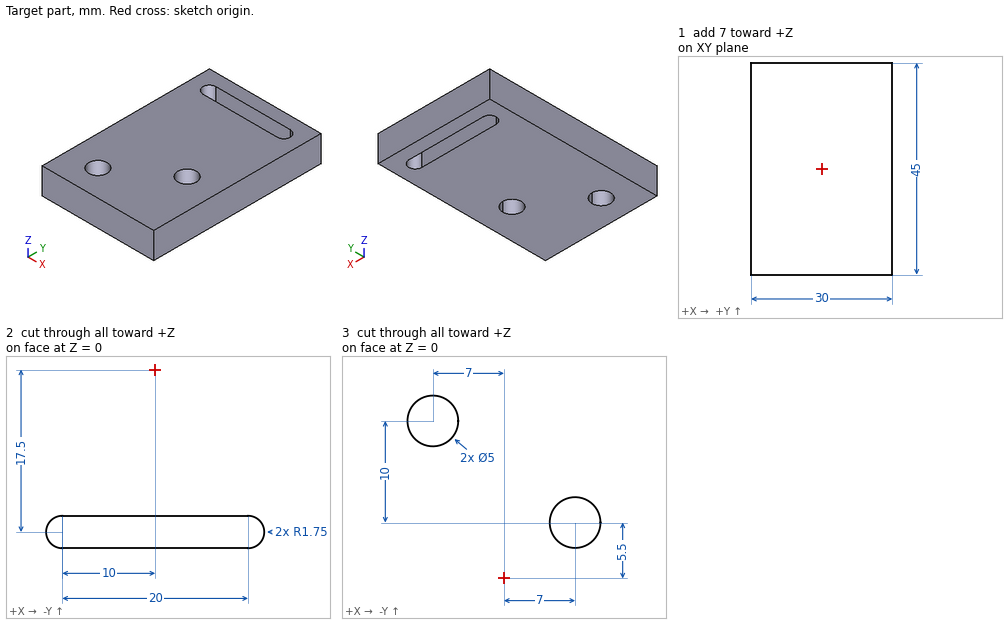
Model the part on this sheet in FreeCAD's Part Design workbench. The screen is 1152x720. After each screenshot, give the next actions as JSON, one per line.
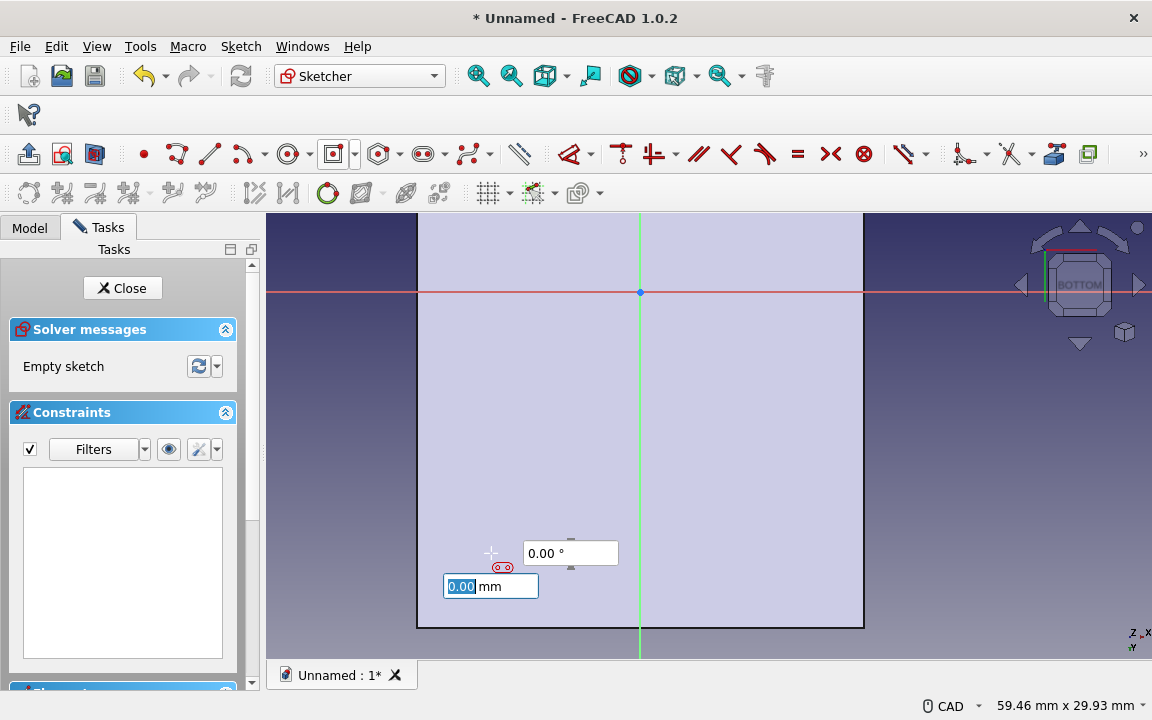
{"action": "left_click", "coordinate": [789, 553]}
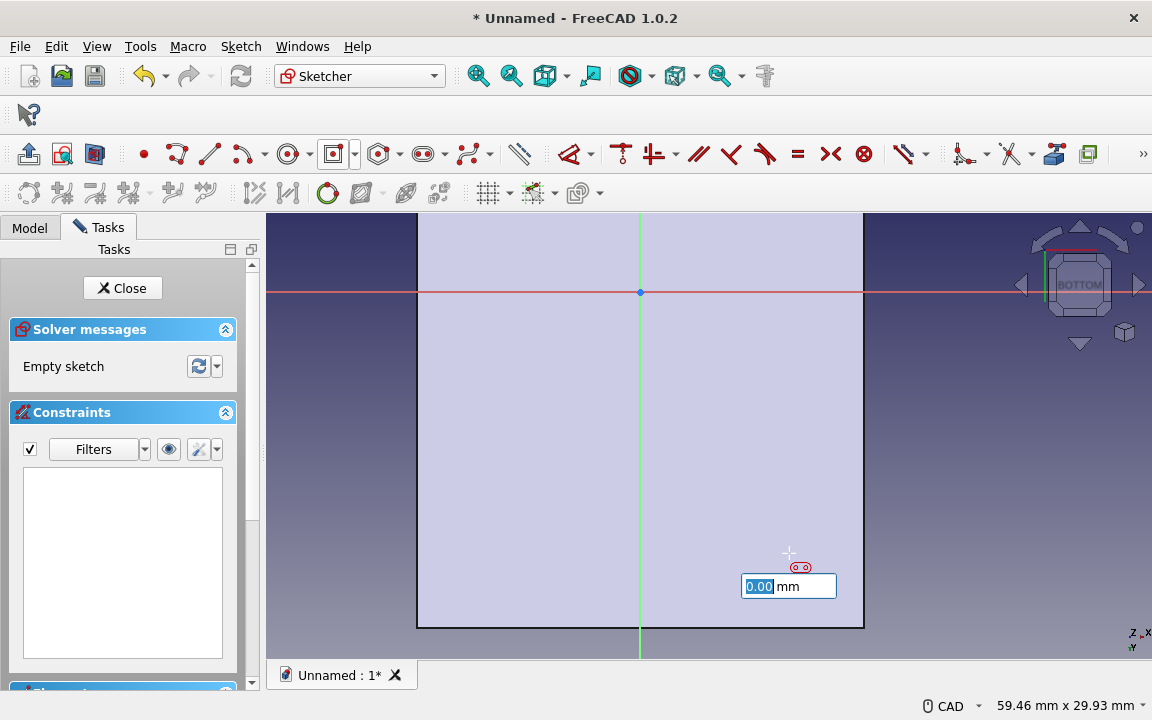
{"action": "left_click", "coordinate": [685, 527]}
{"action": "key", "text": "Escape"}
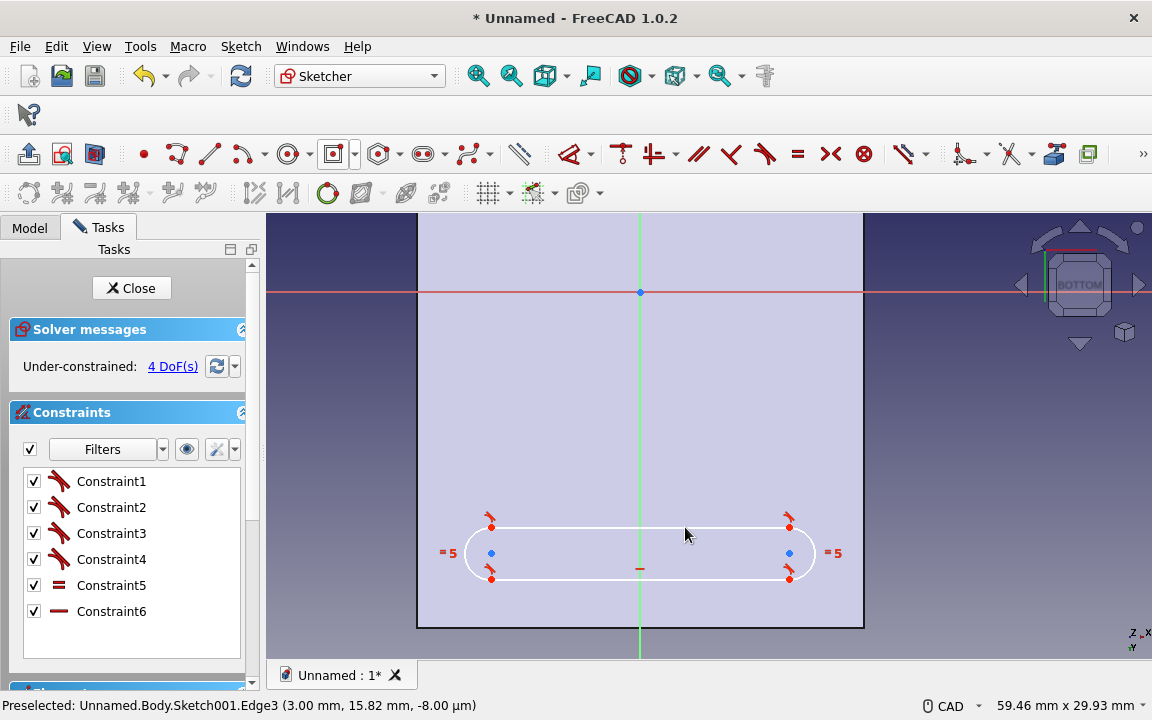
{"action": "left_click", "coordinate": [568, 154]}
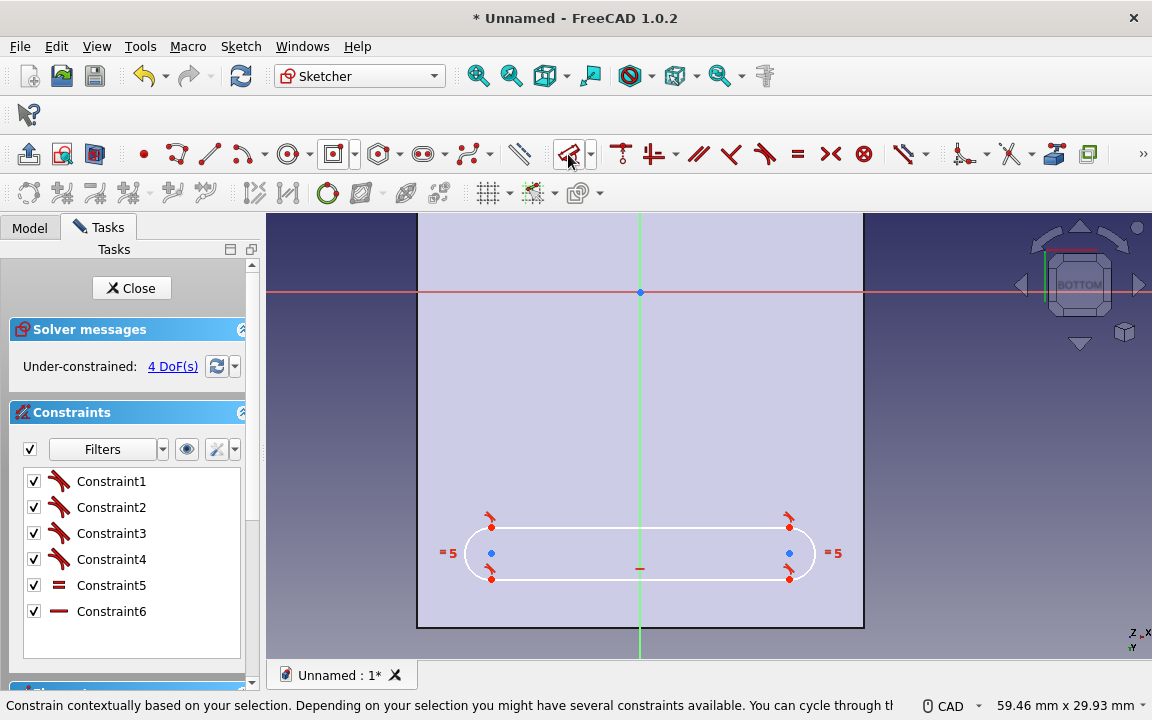
{"action": "scroll", "coordinate": [470, 539], "scroll_direction": "up", "scroll_amount": 3}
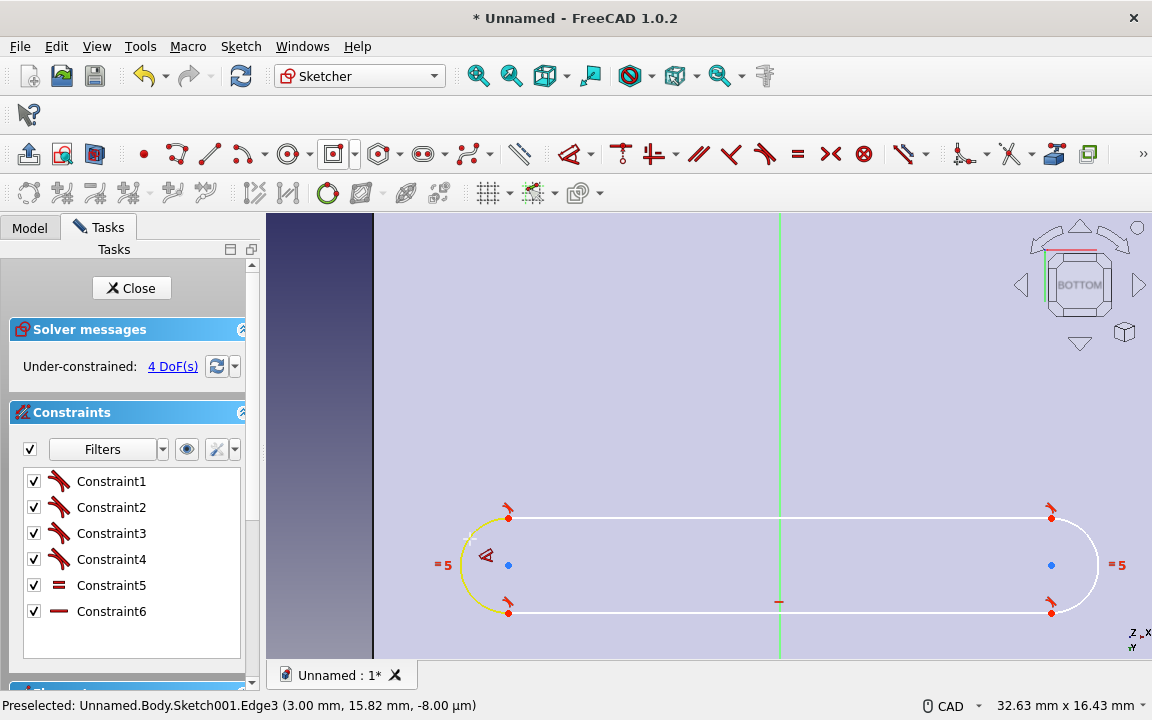
{"action": "left_click", "coordinate": [470, 538]}
{"action": "left_click", "coordinate": [444, 519]}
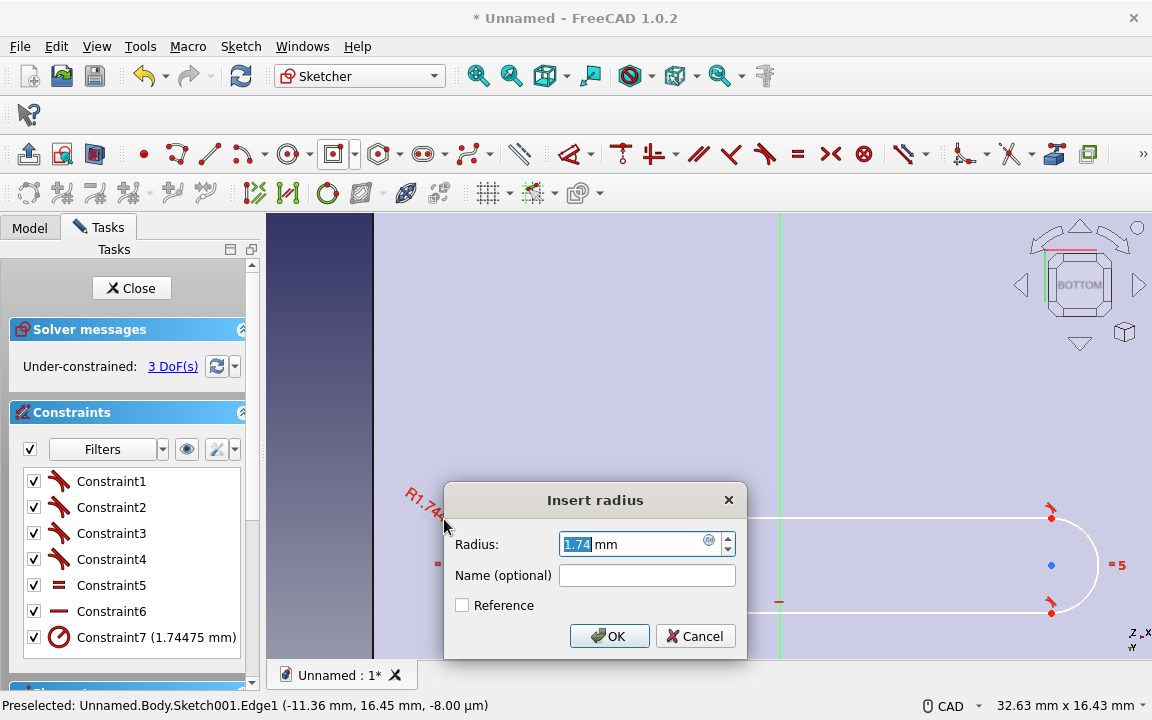
{"action": "type", "text": "1.75"}
{"action": "key", "text": "Return"}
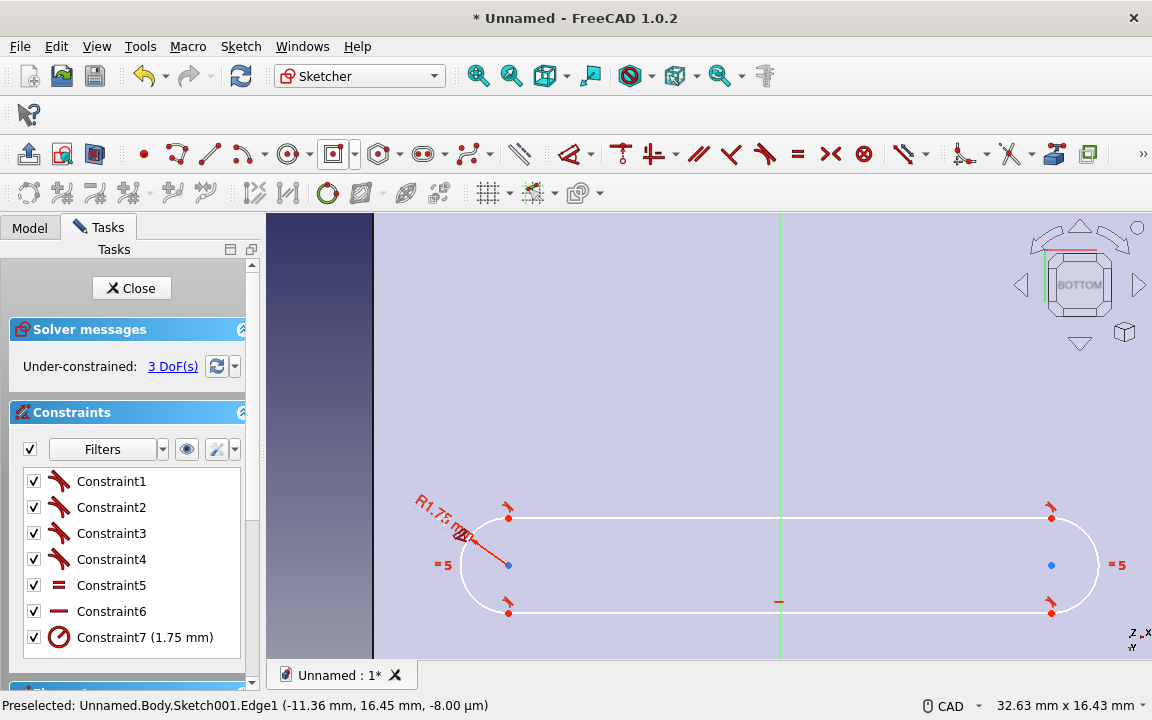
{"action": "left_click", "coordinate": [671, 518]}
{"action": "left_click", "coordinate": [748, 552]}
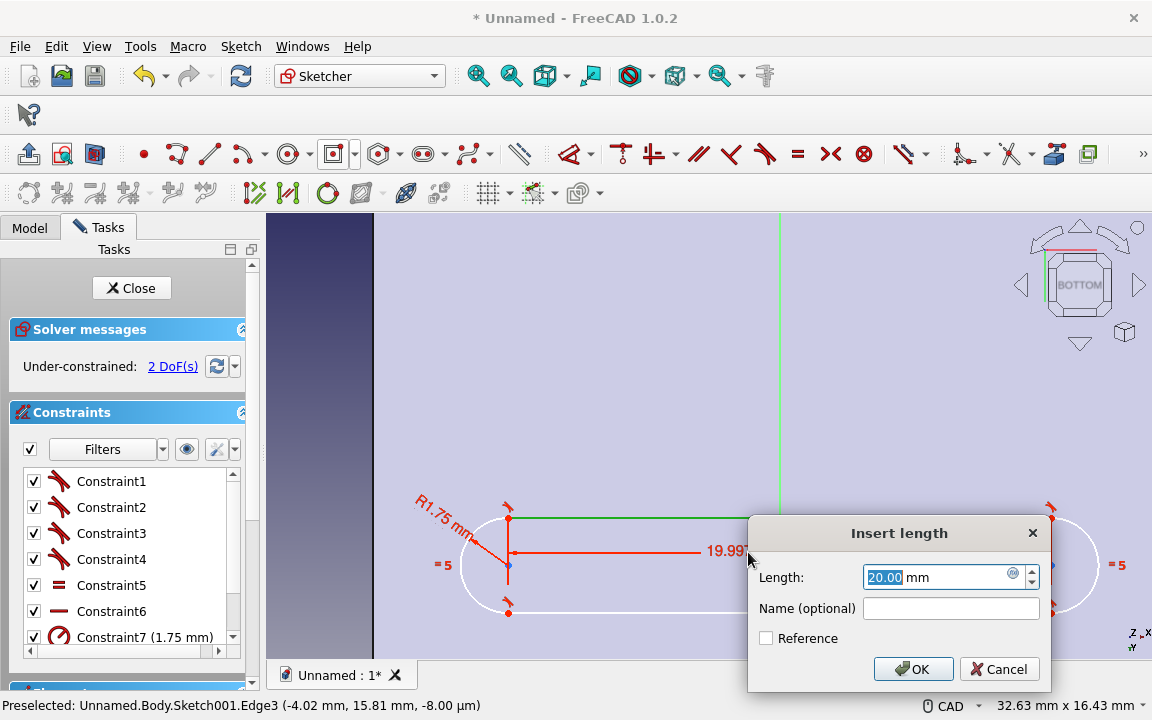
{"action": "type", "text": "20"}
{"action": "key", "text": "Return"}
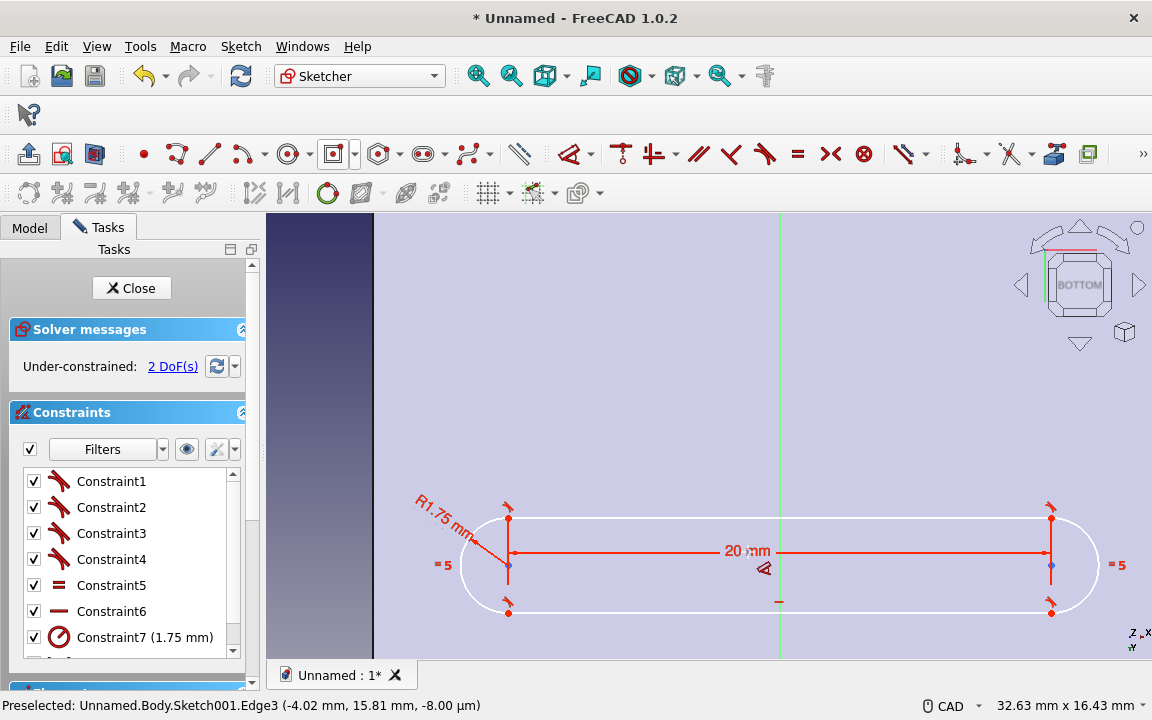
{"action": "left_click", "coordinate": [508, 518]}
{"action": "left_click", "coordinate": [644, 552]}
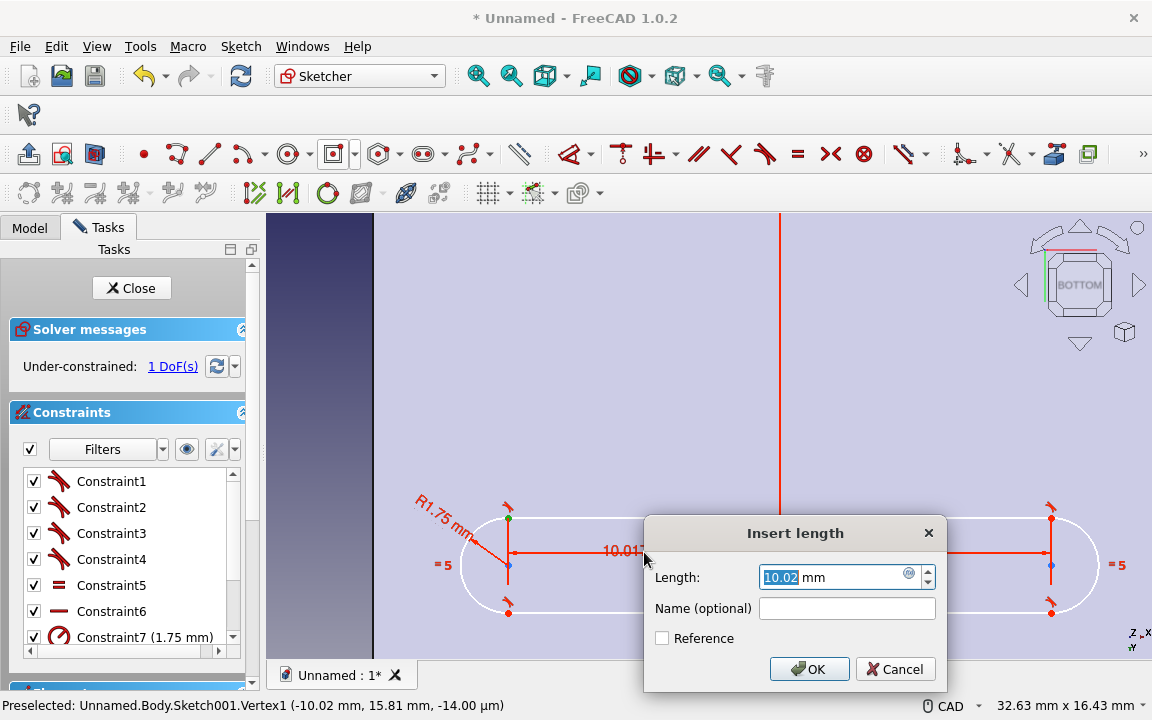
{"action": "type", "text": "10"}
{"action": "key", "text": "Return"}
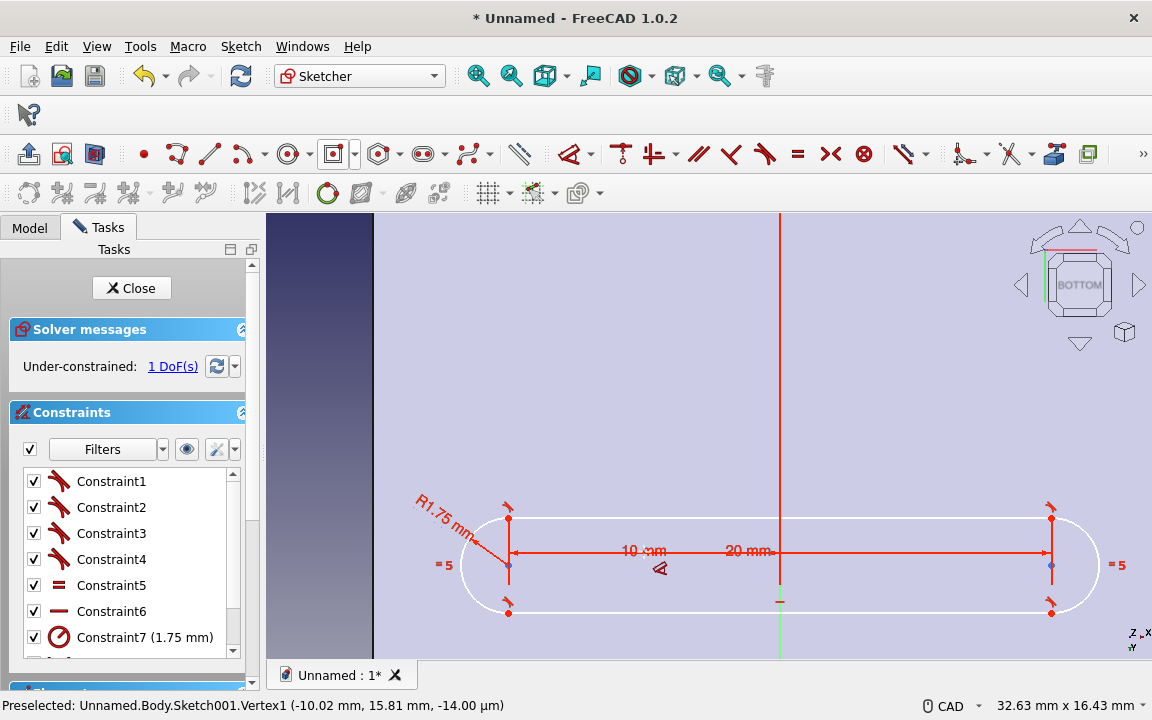
{"action": "left_click", "coordinate": [509, 566]}
{"action": "left_click", "coordinate": [475, 403]}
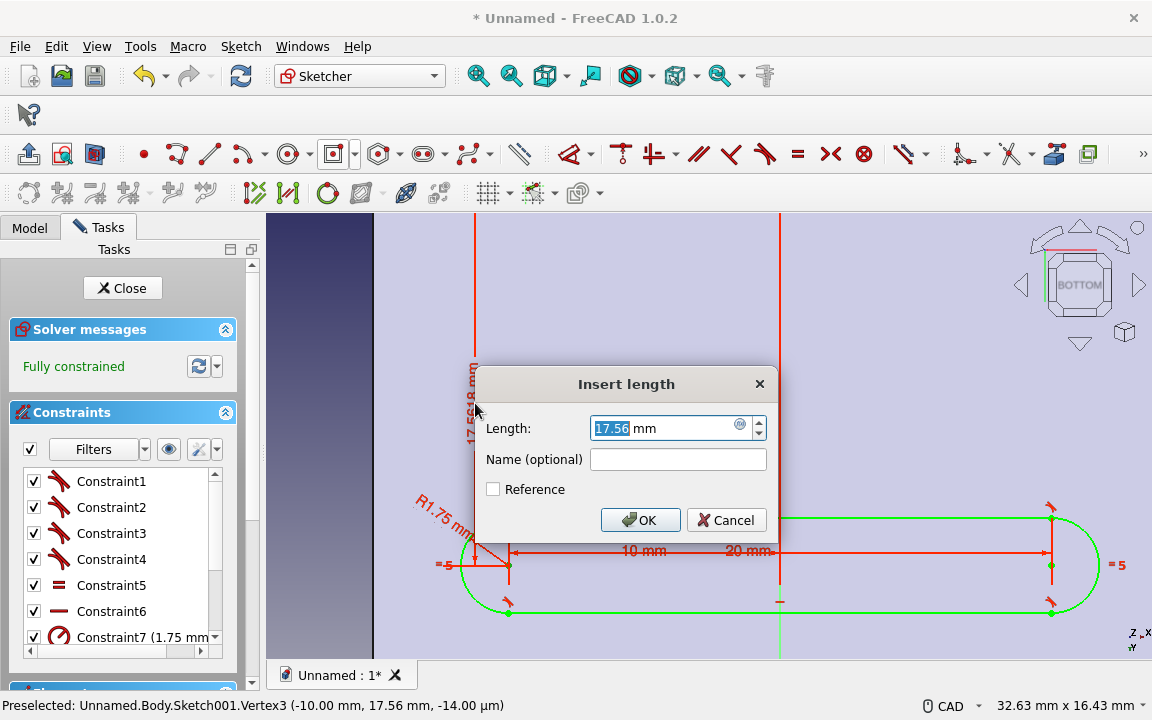
{"action": "type", "text": "17.5"}
{"action": "key", "text": "Return"}
{"action": "key", "text": "Escape"}